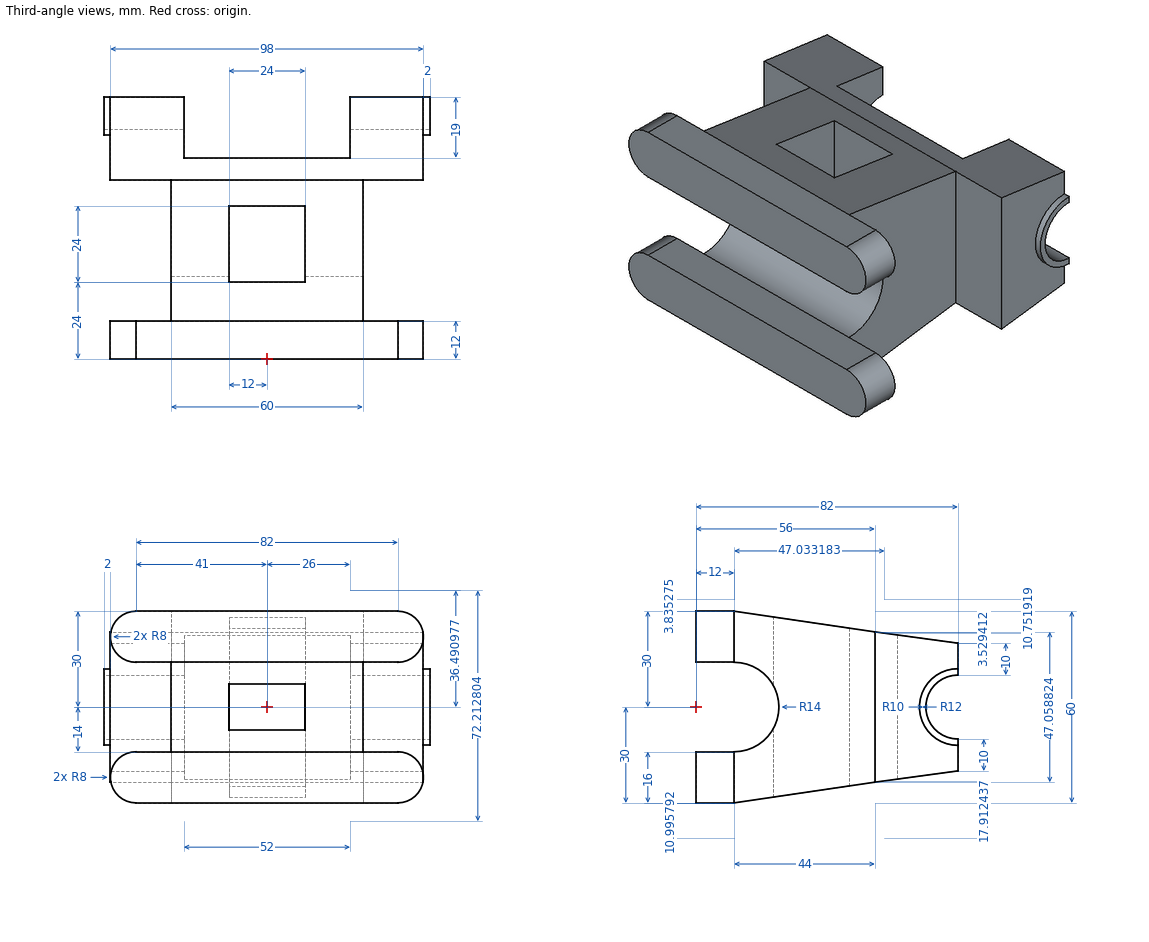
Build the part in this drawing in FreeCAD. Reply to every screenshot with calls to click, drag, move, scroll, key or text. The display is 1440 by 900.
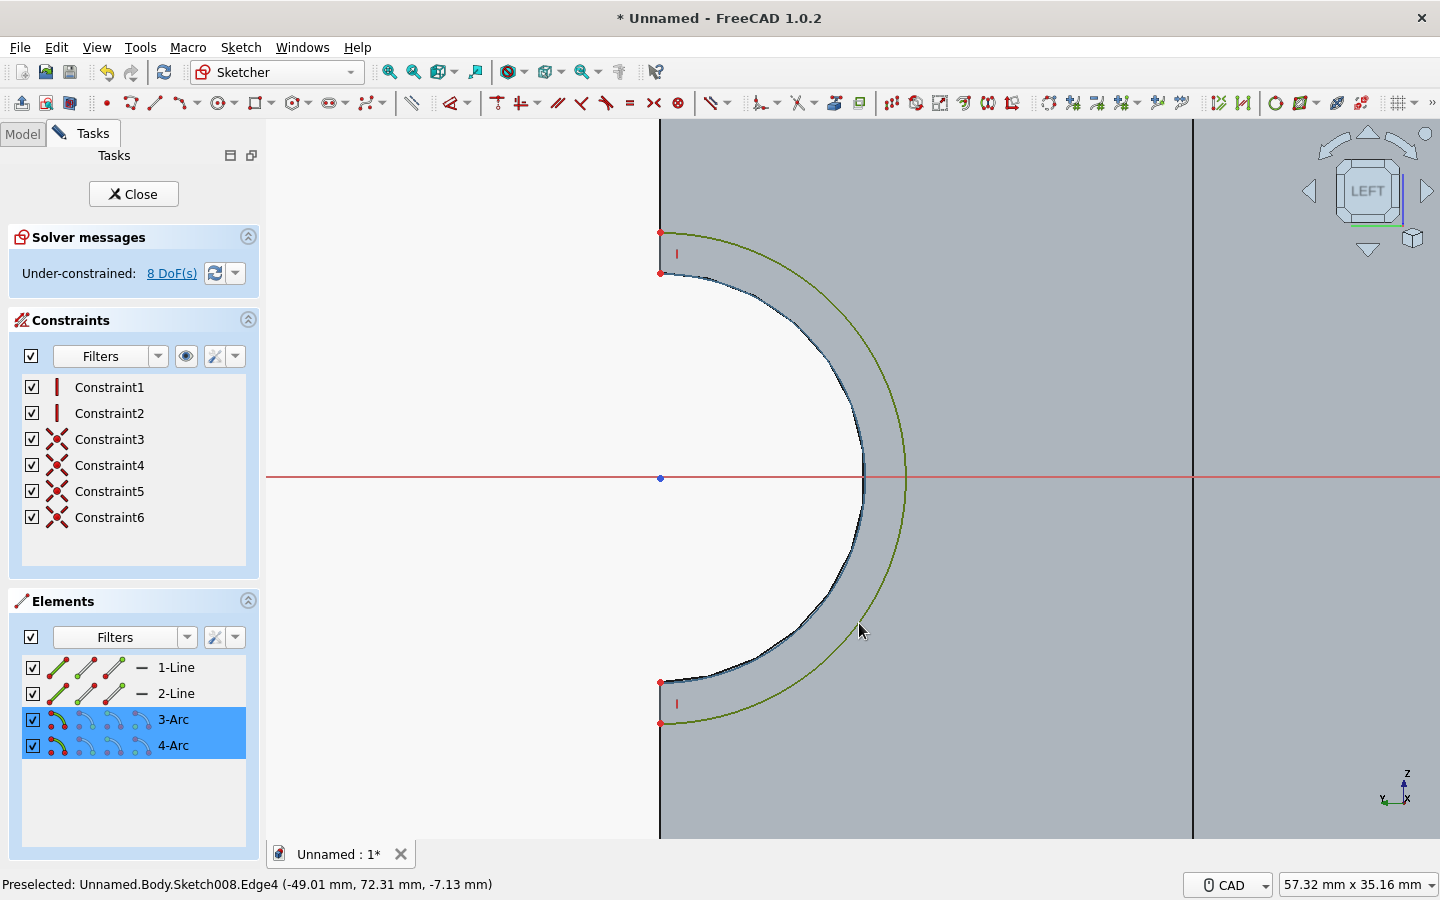
click(498, 104)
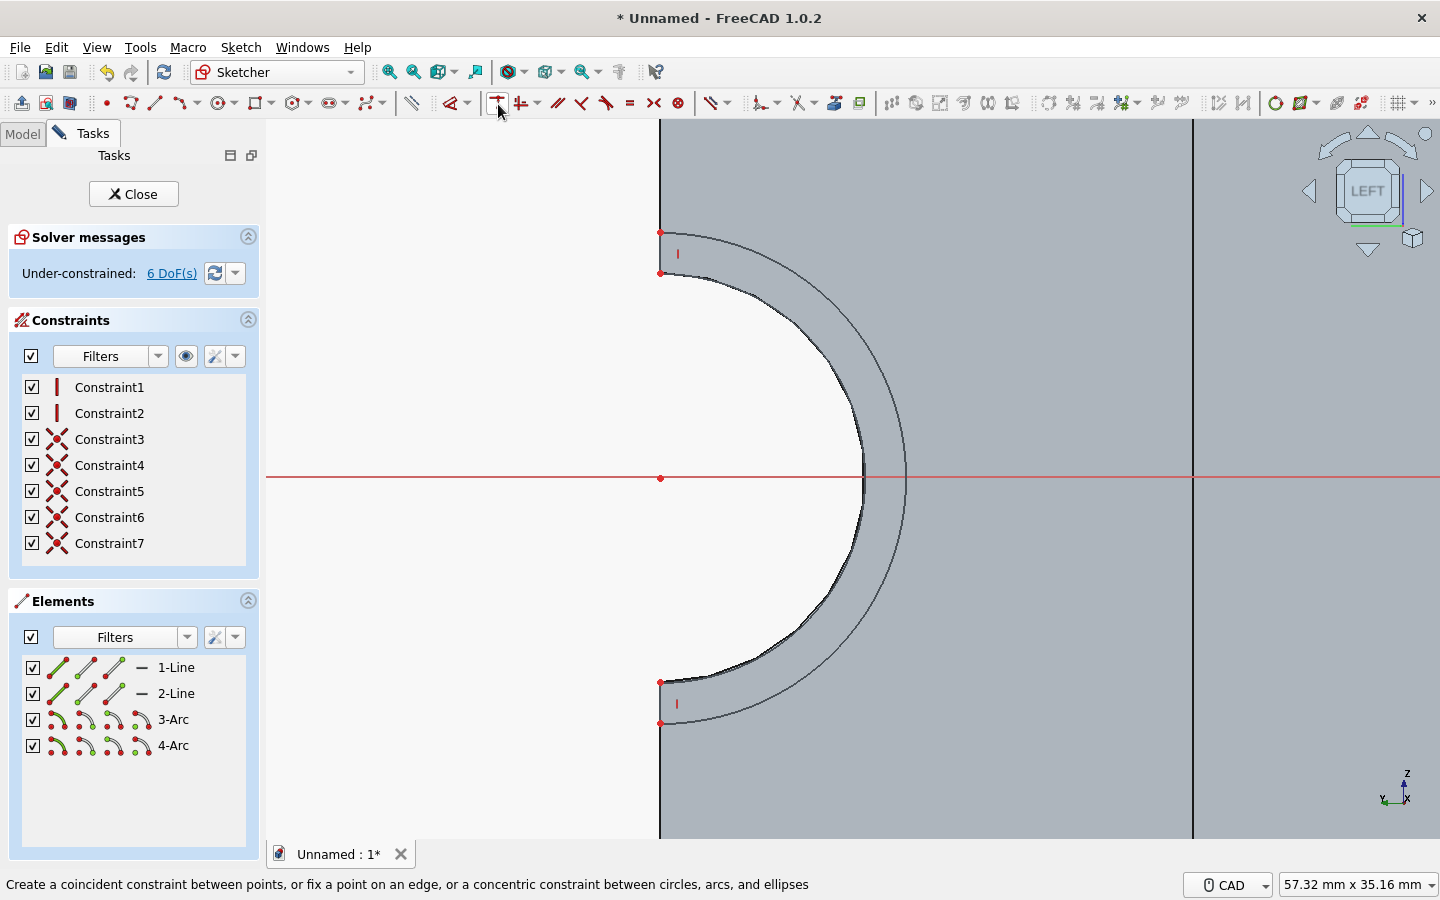
click(661, 479)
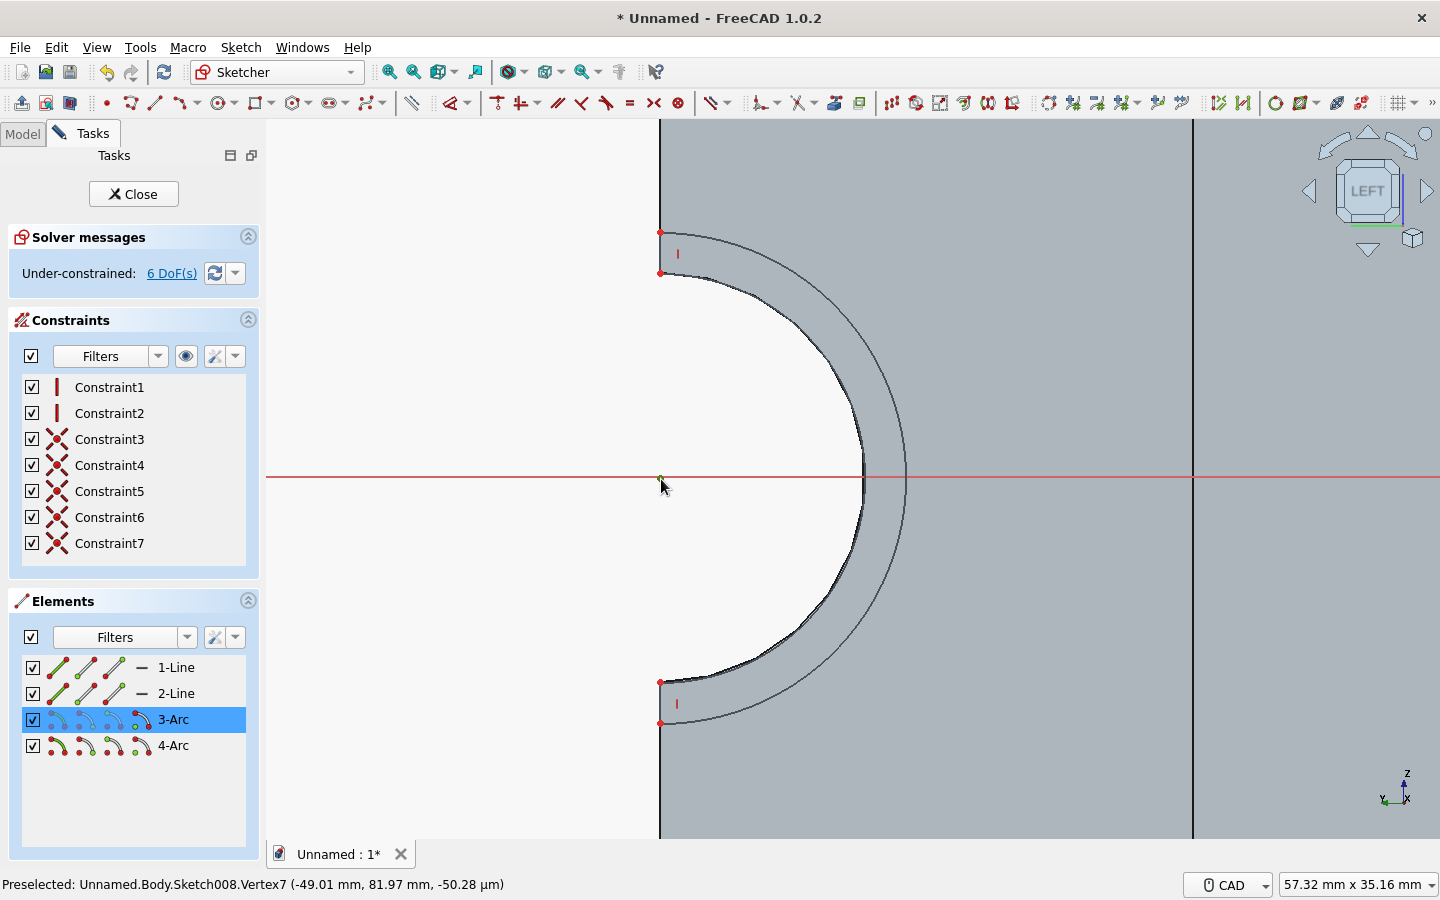
click(364, 477)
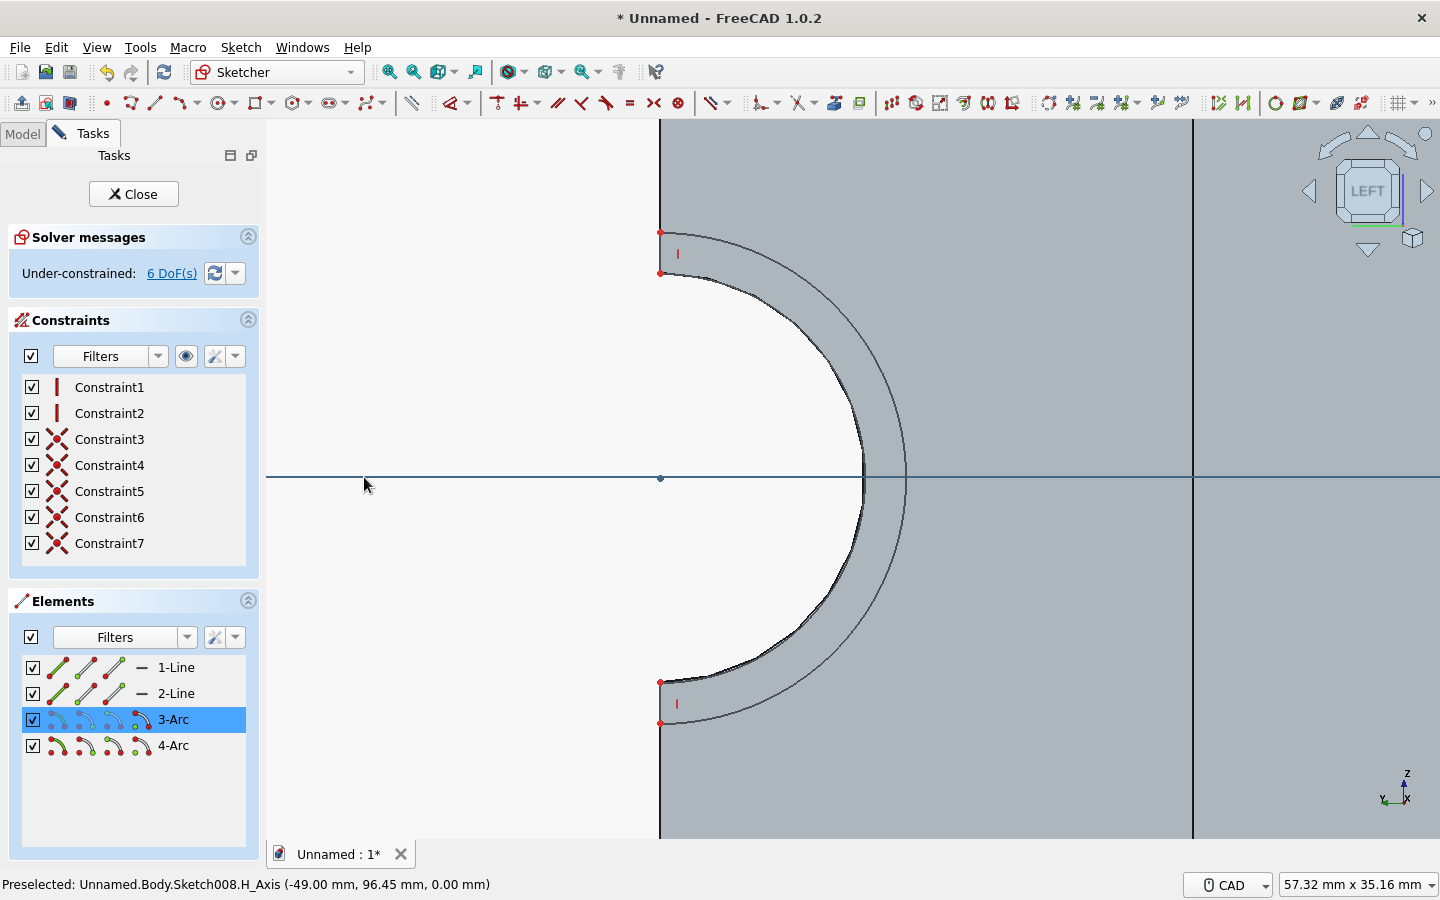
click(498, 104)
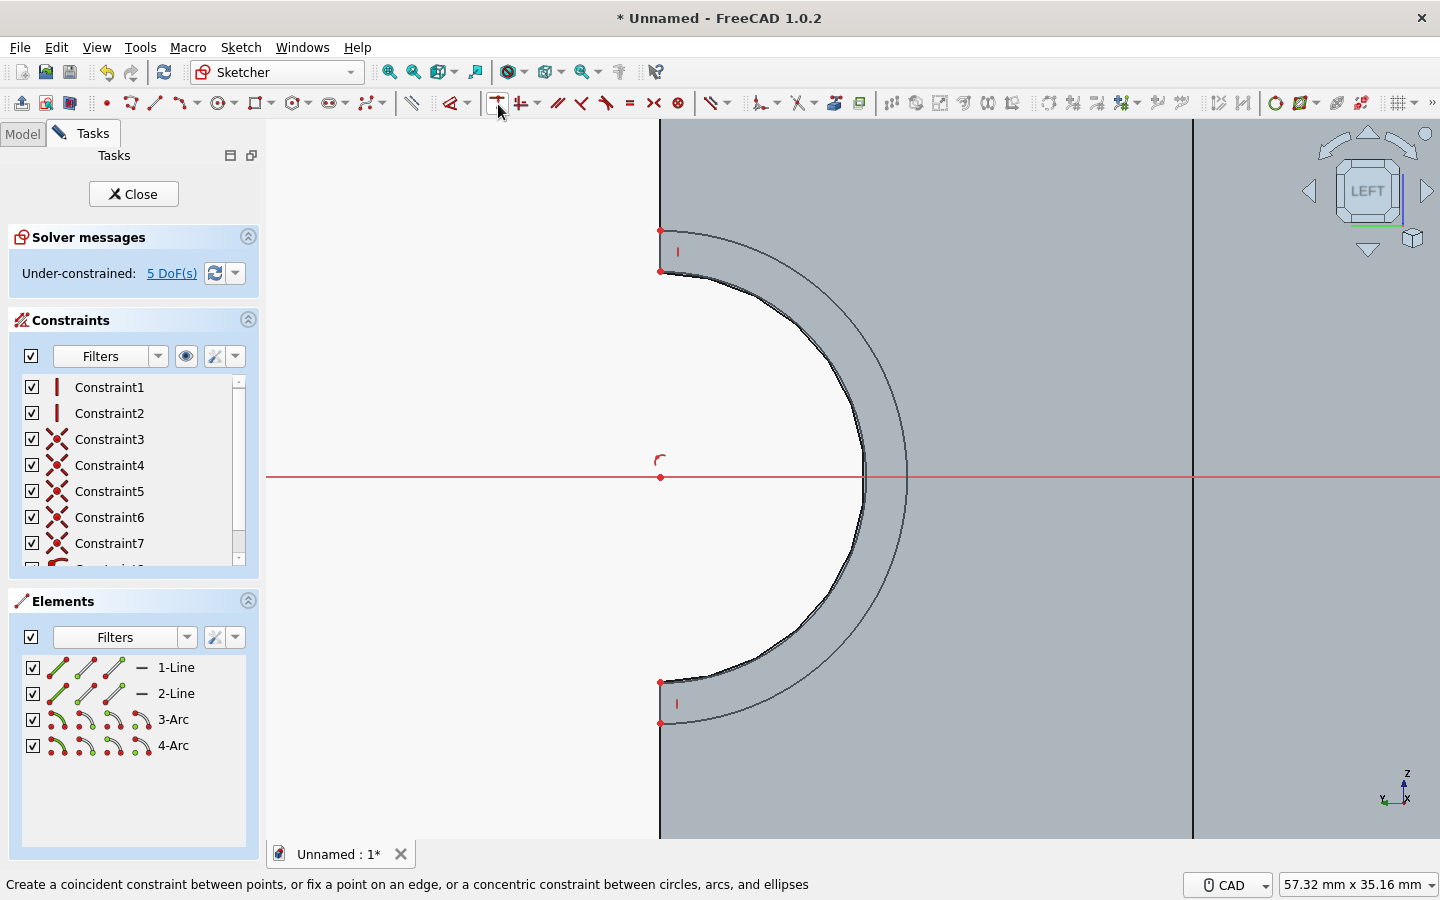
click(450, 104)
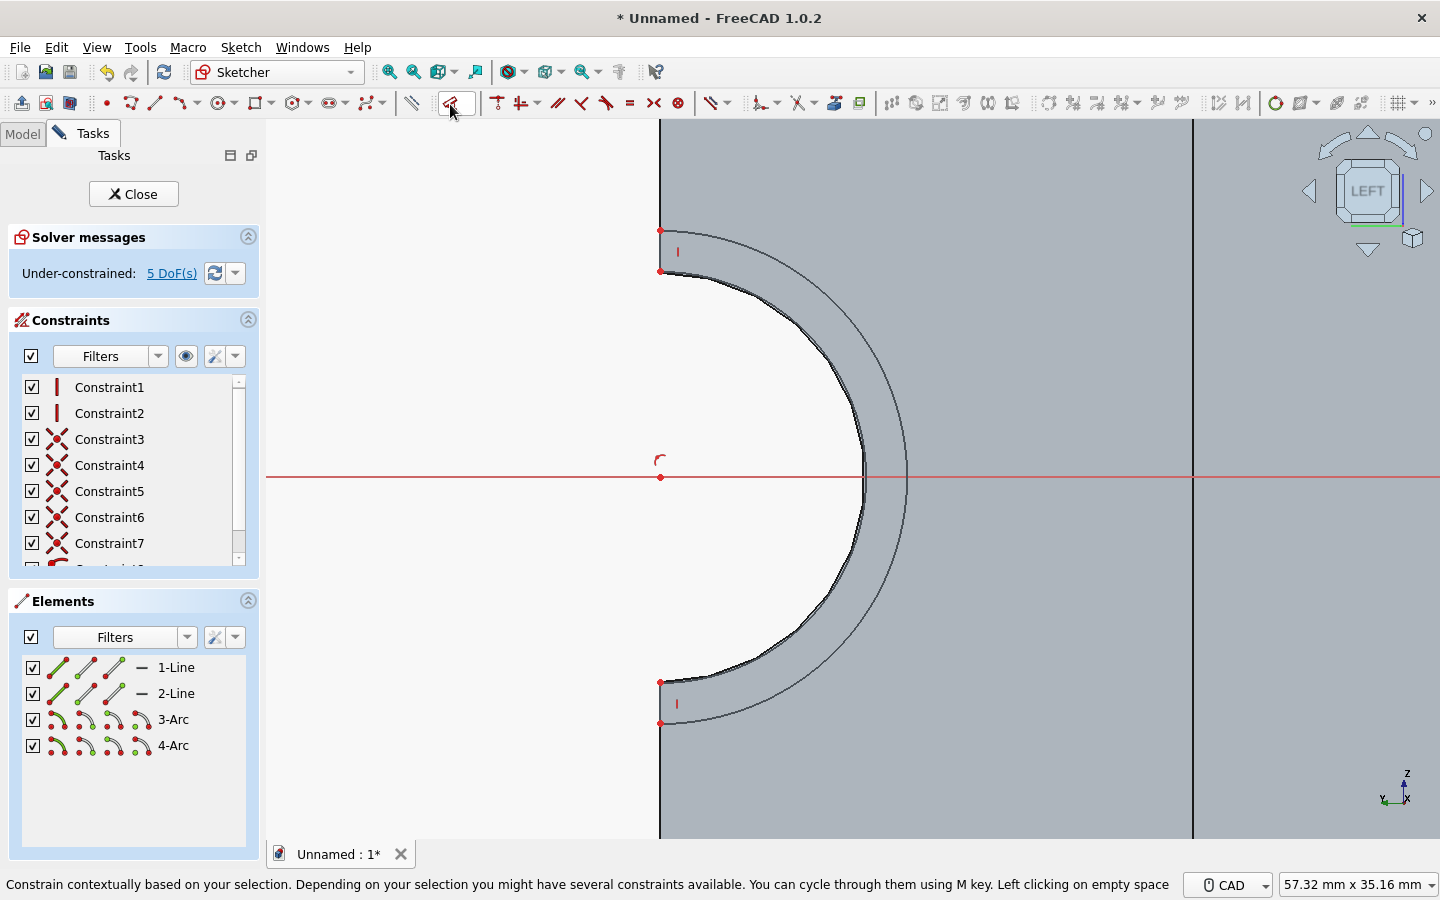
click(827, 598)
click(521, 670)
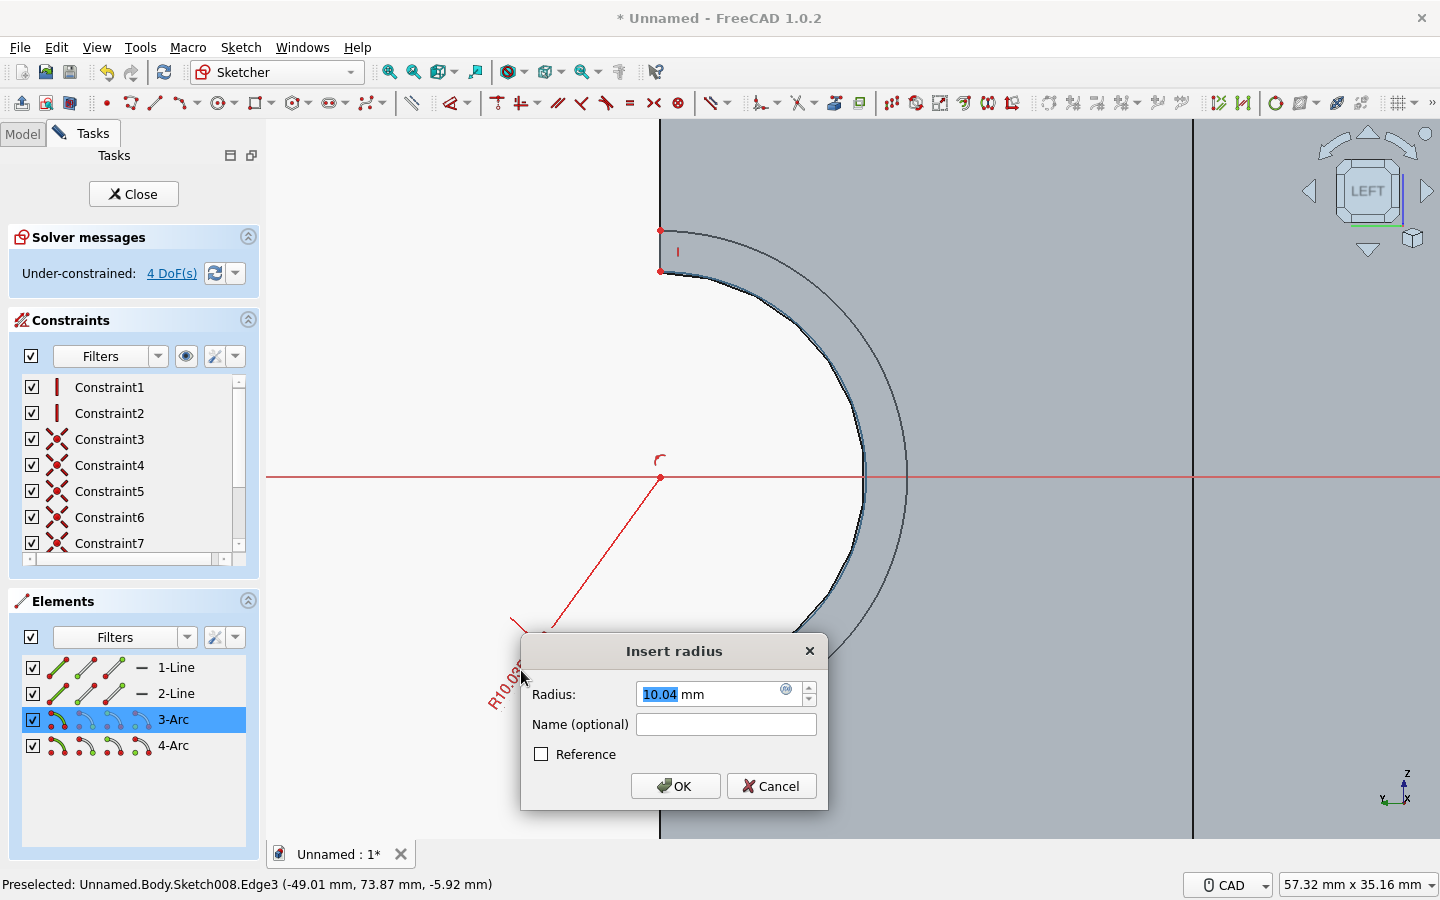
text(10)
key(Return)